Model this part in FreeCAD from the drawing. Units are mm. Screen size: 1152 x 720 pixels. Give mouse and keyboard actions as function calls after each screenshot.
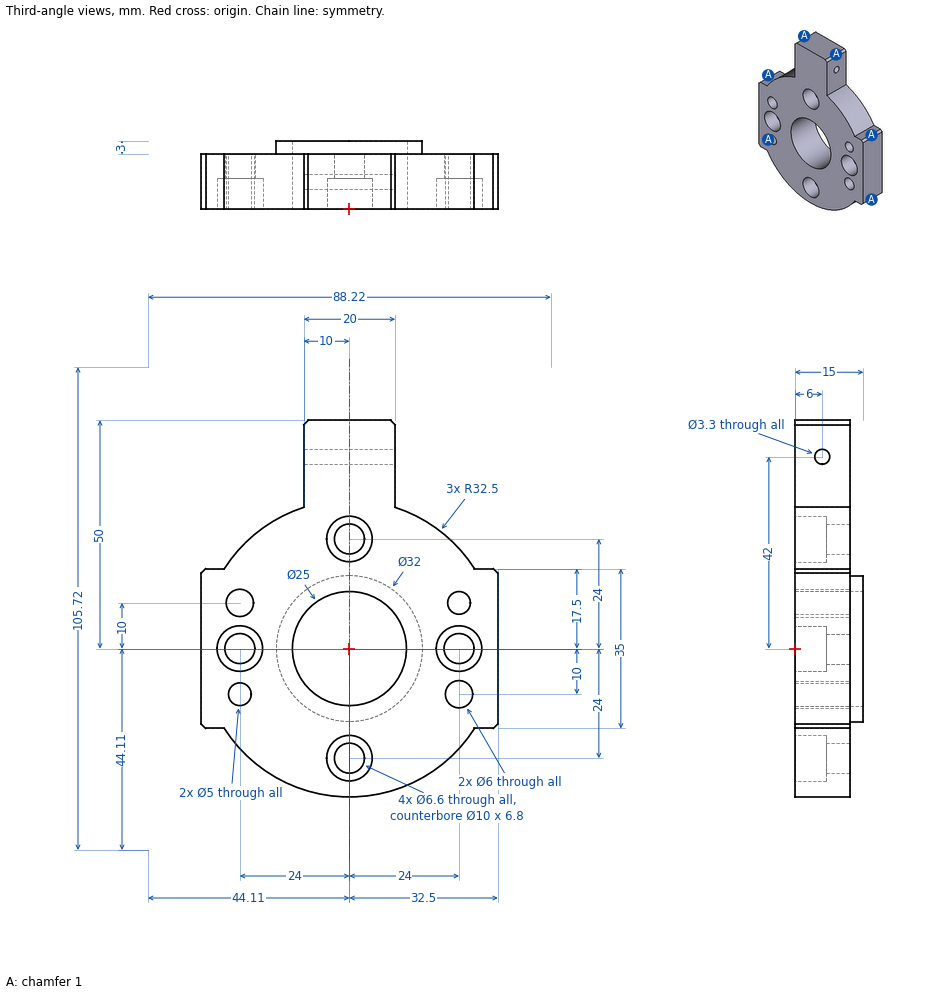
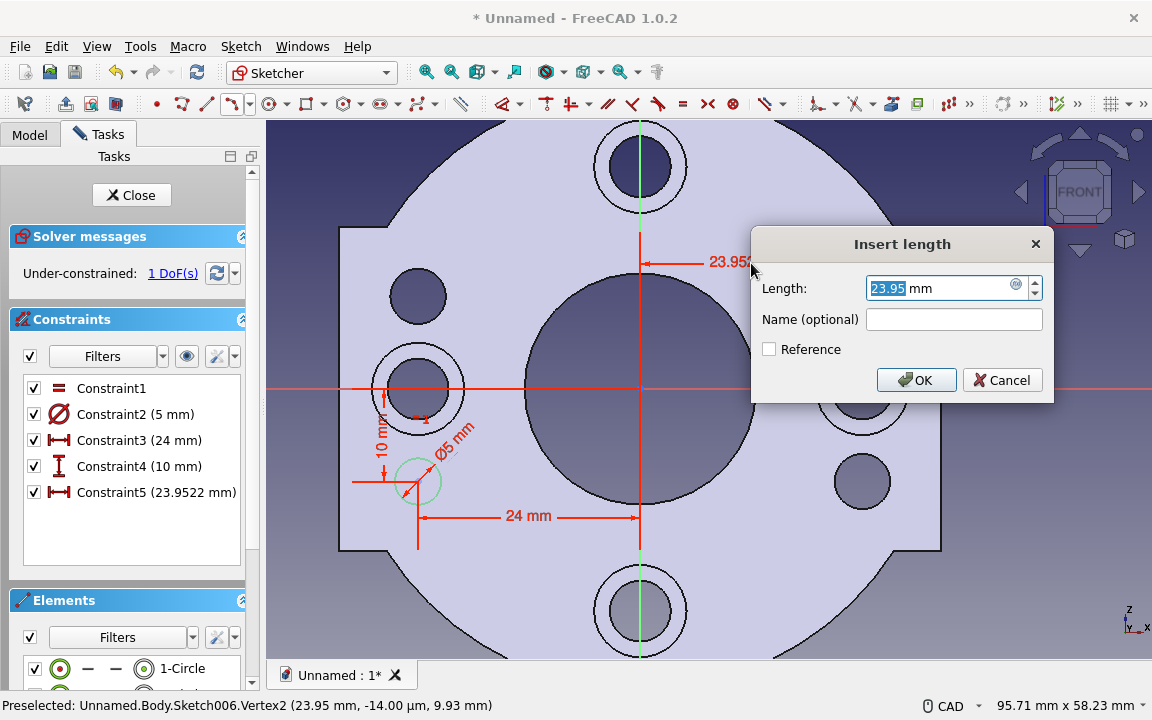
text(24)
key(Return)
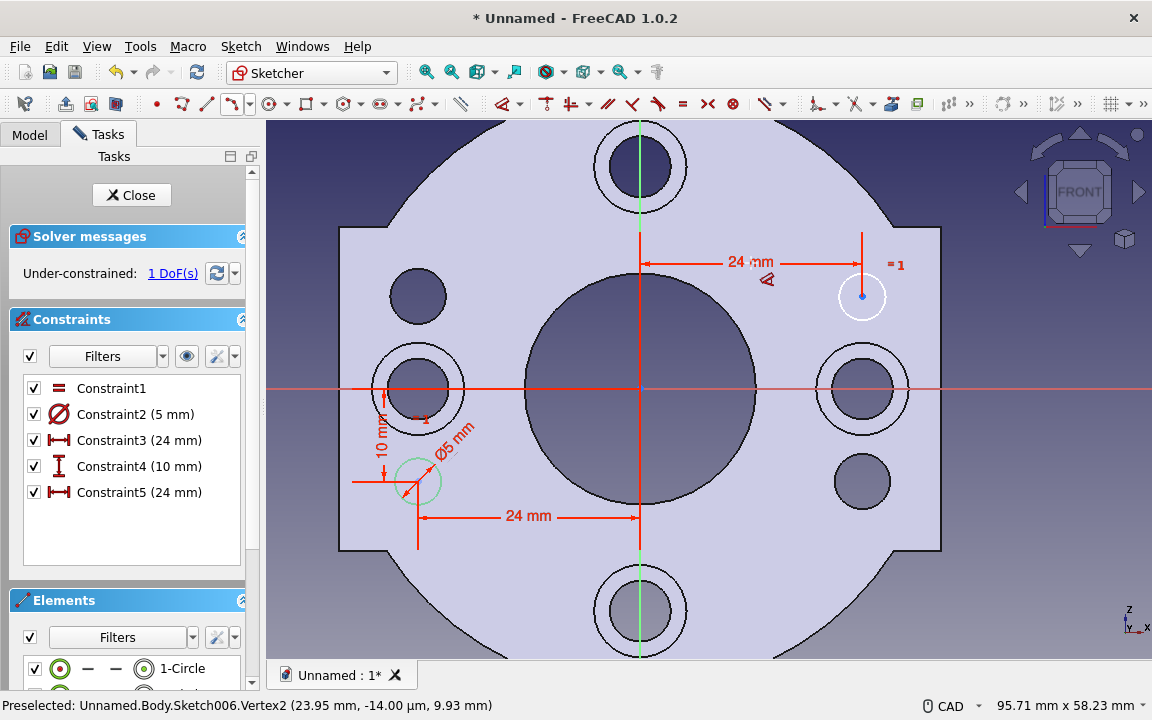
click(862, 297)
click(896, 343)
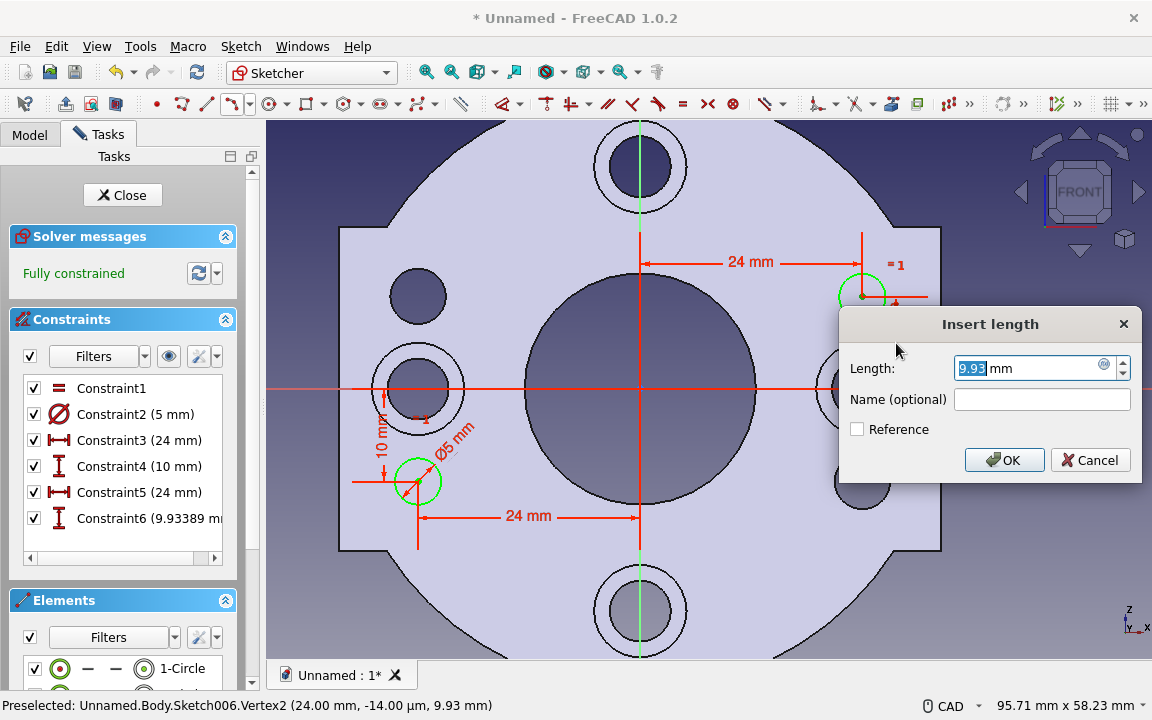
text(10)
key(Return)
key(Escape)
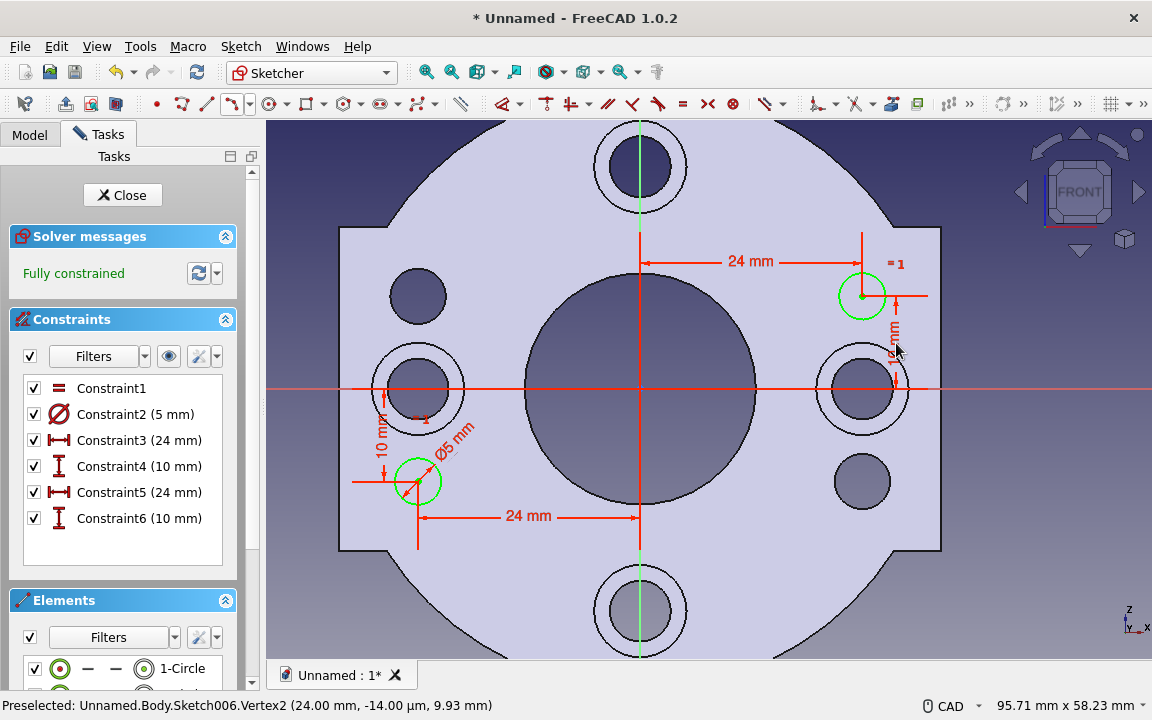
click(123, 195)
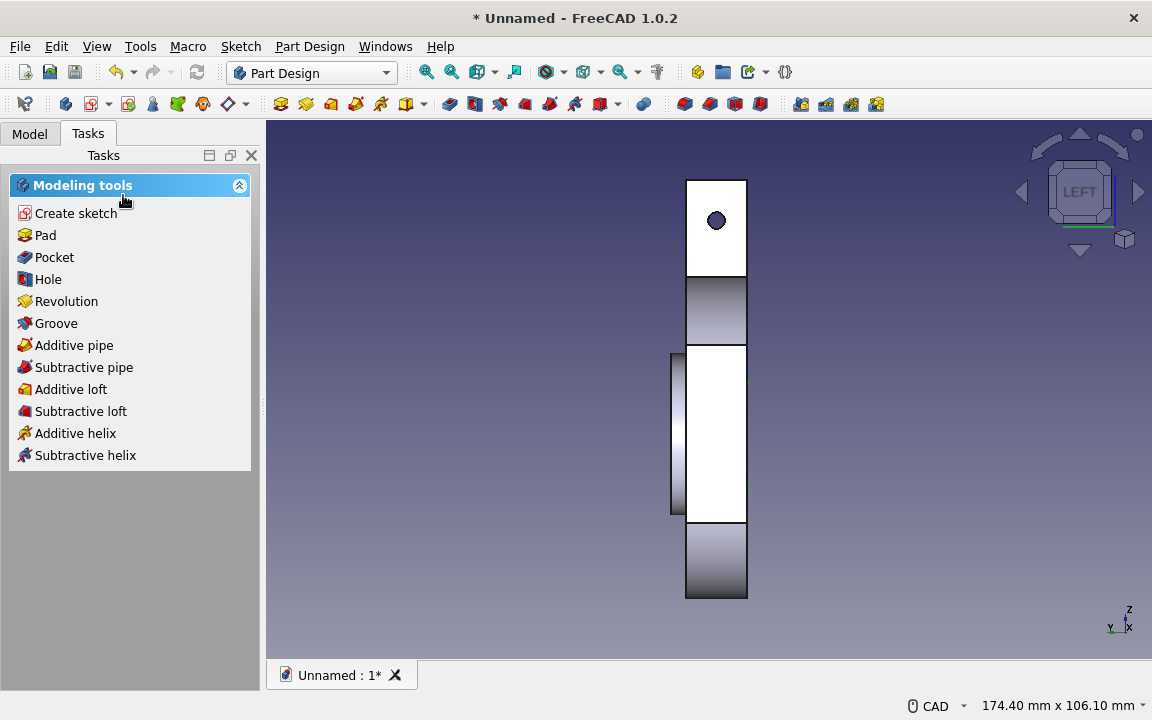
click(475, 104)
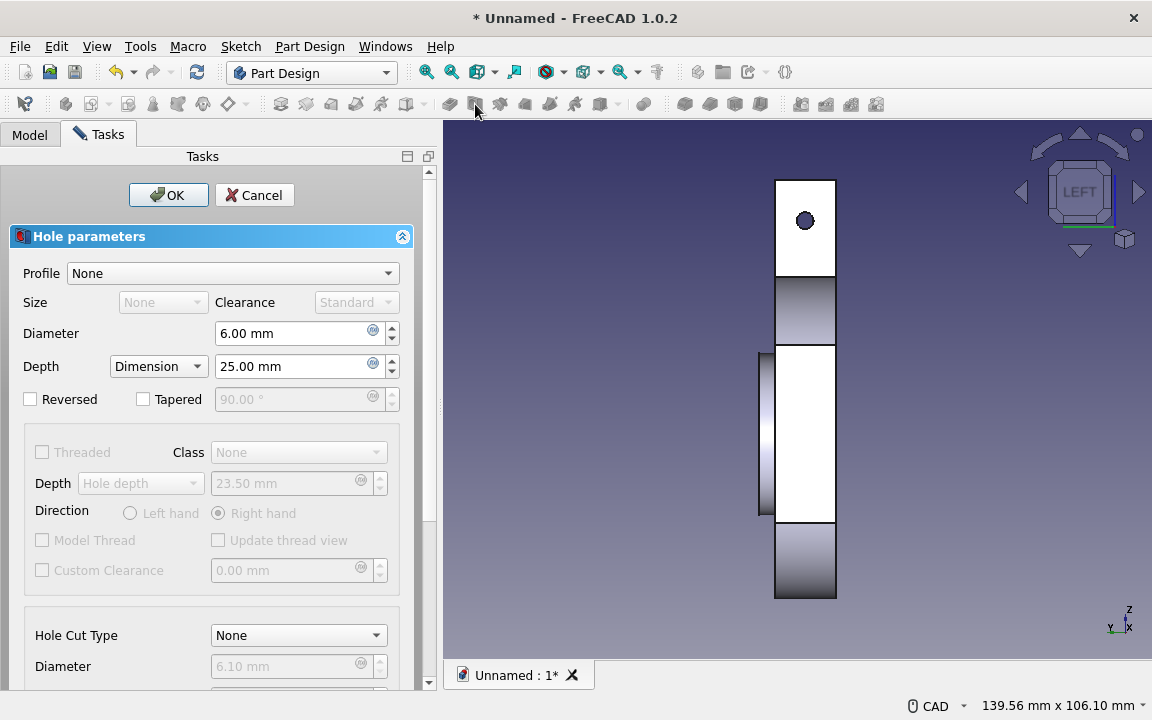
triple_click(300, 334)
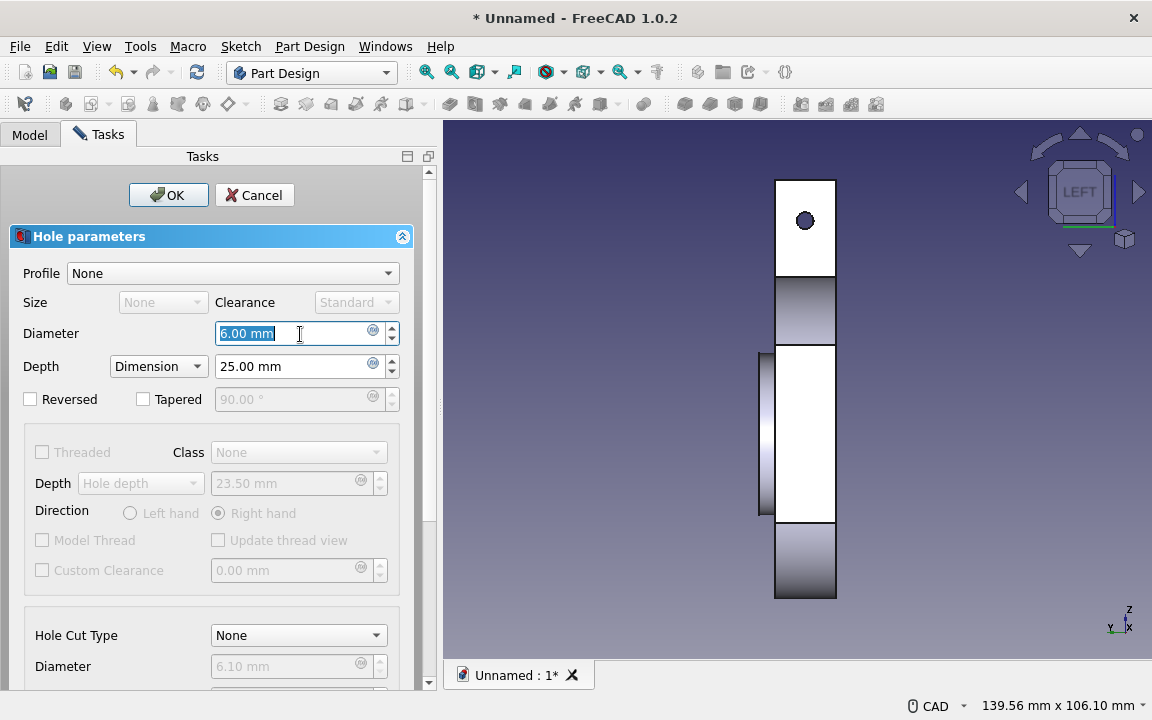
text(5)
key(Tab)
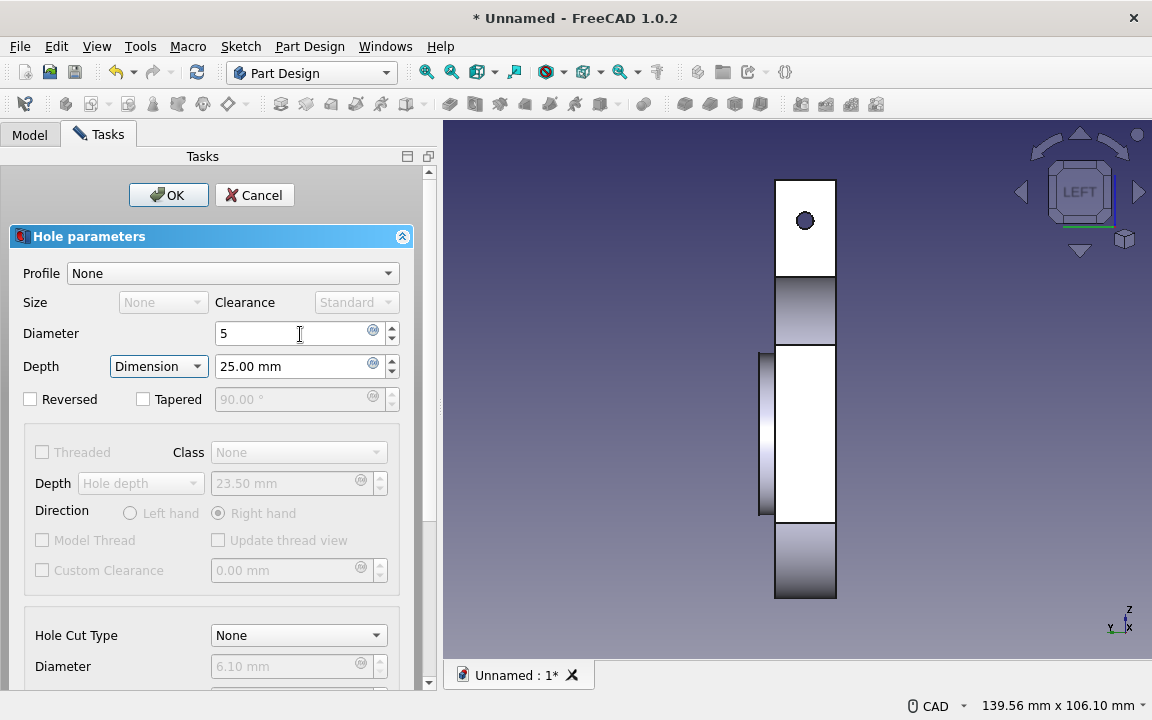
click(160, 366)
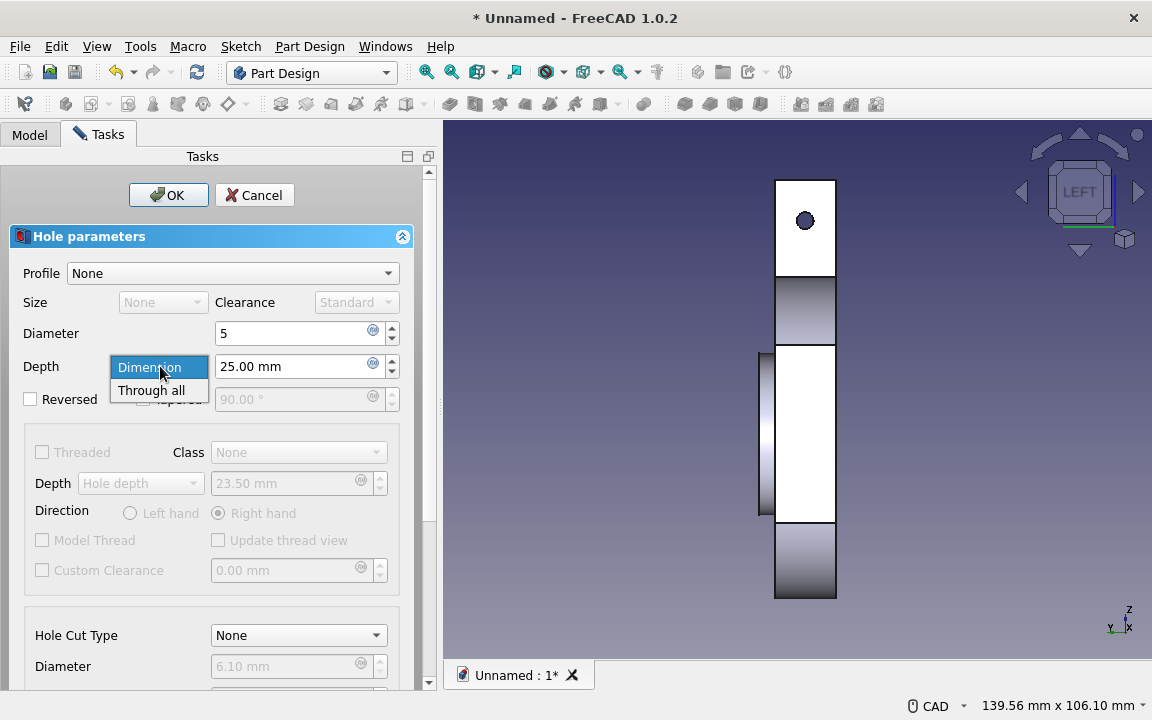
click(158, 390)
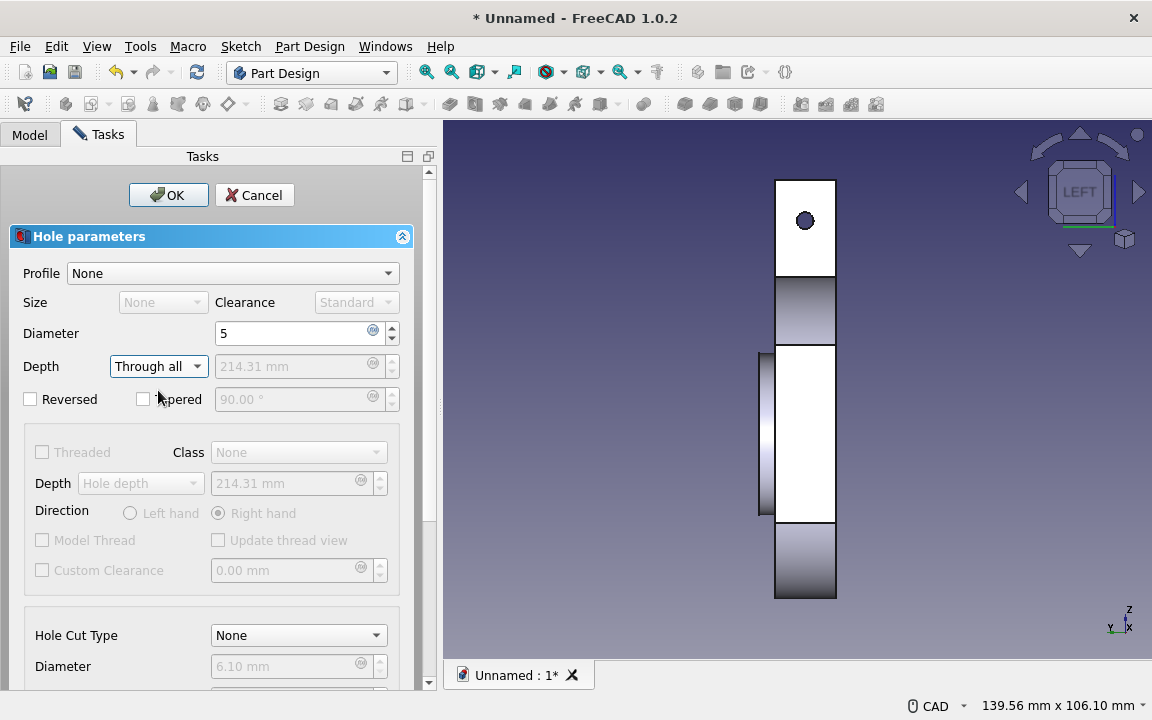
click(169, 195)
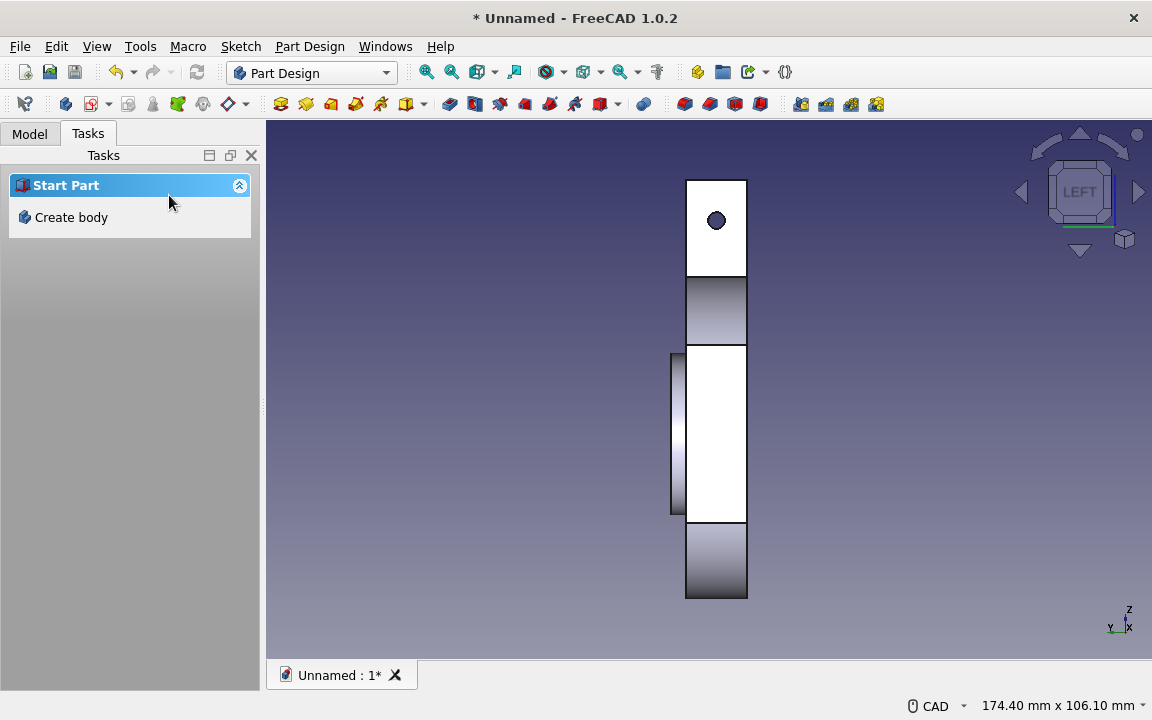
click(717, 179)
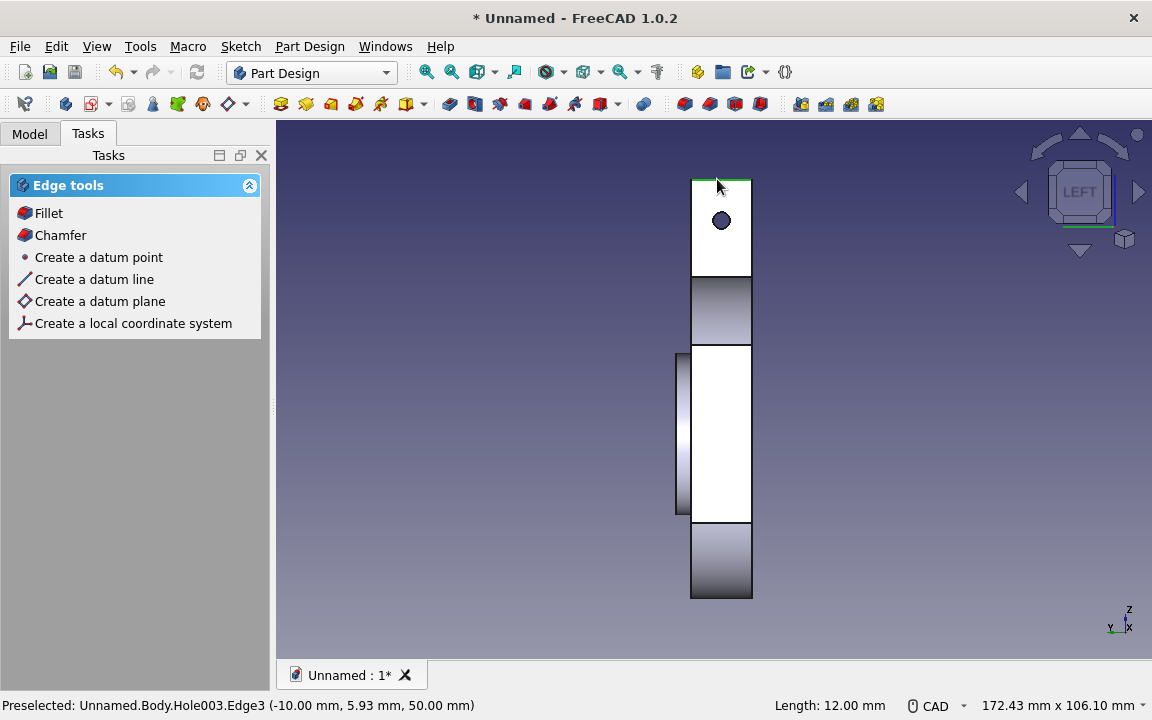
click(722, 344, ctrl)